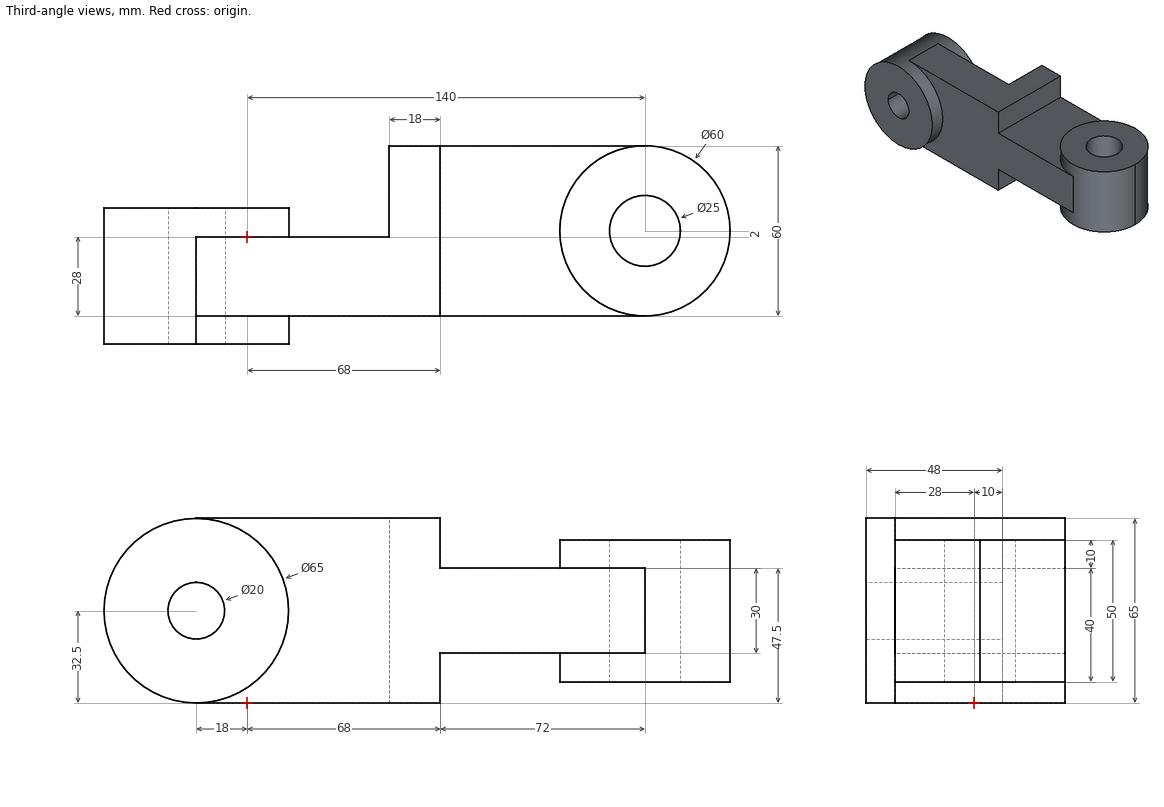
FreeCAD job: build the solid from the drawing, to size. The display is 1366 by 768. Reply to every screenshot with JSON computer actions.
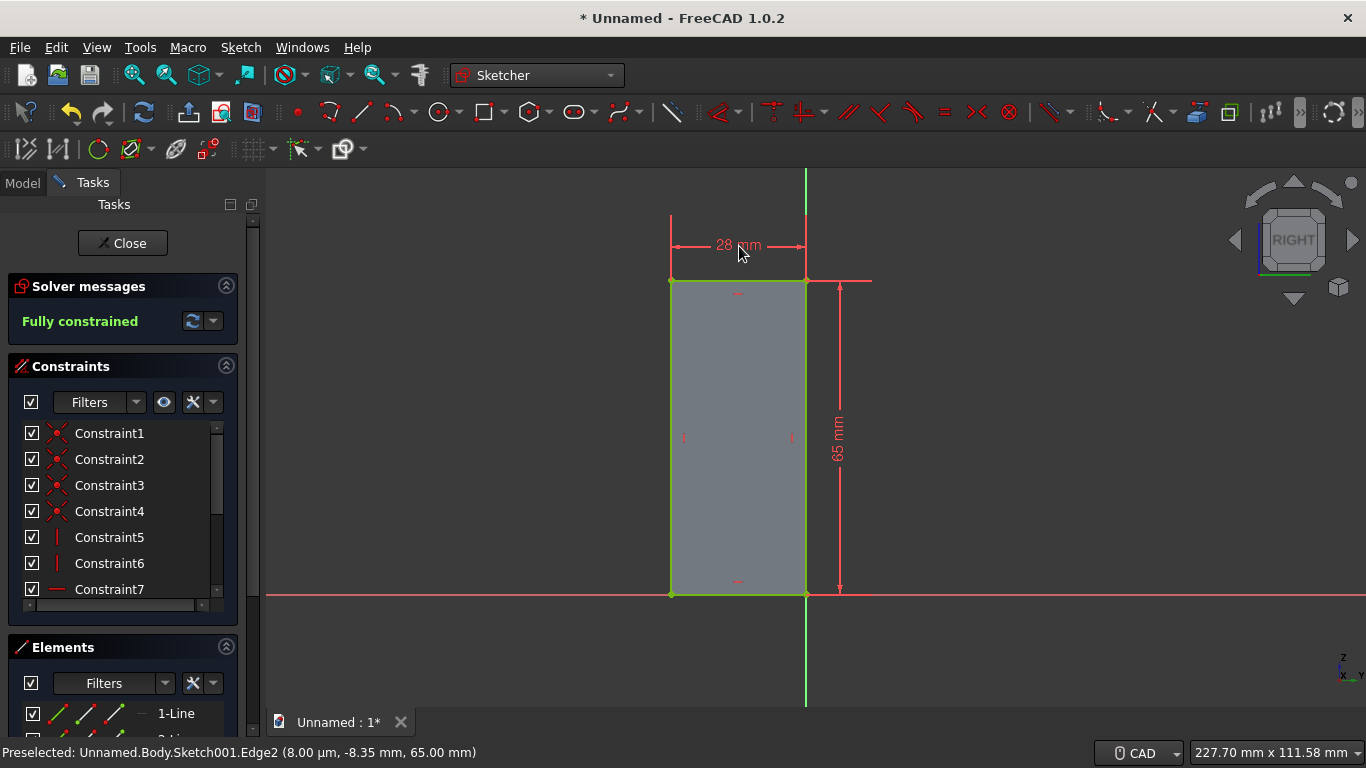
{"action": "left_click", "coordinate": [123, 243]}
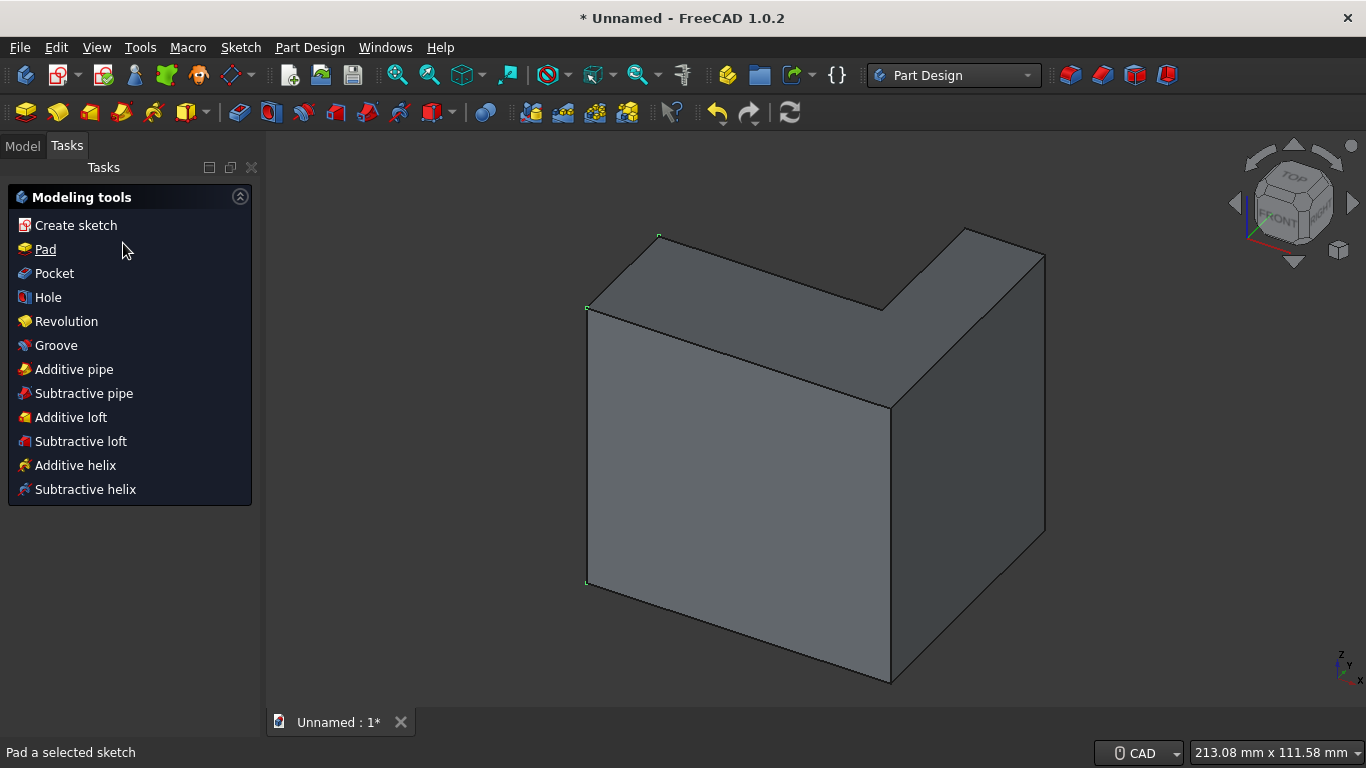
{"action": "left_click", "coordinate": [26, 112]}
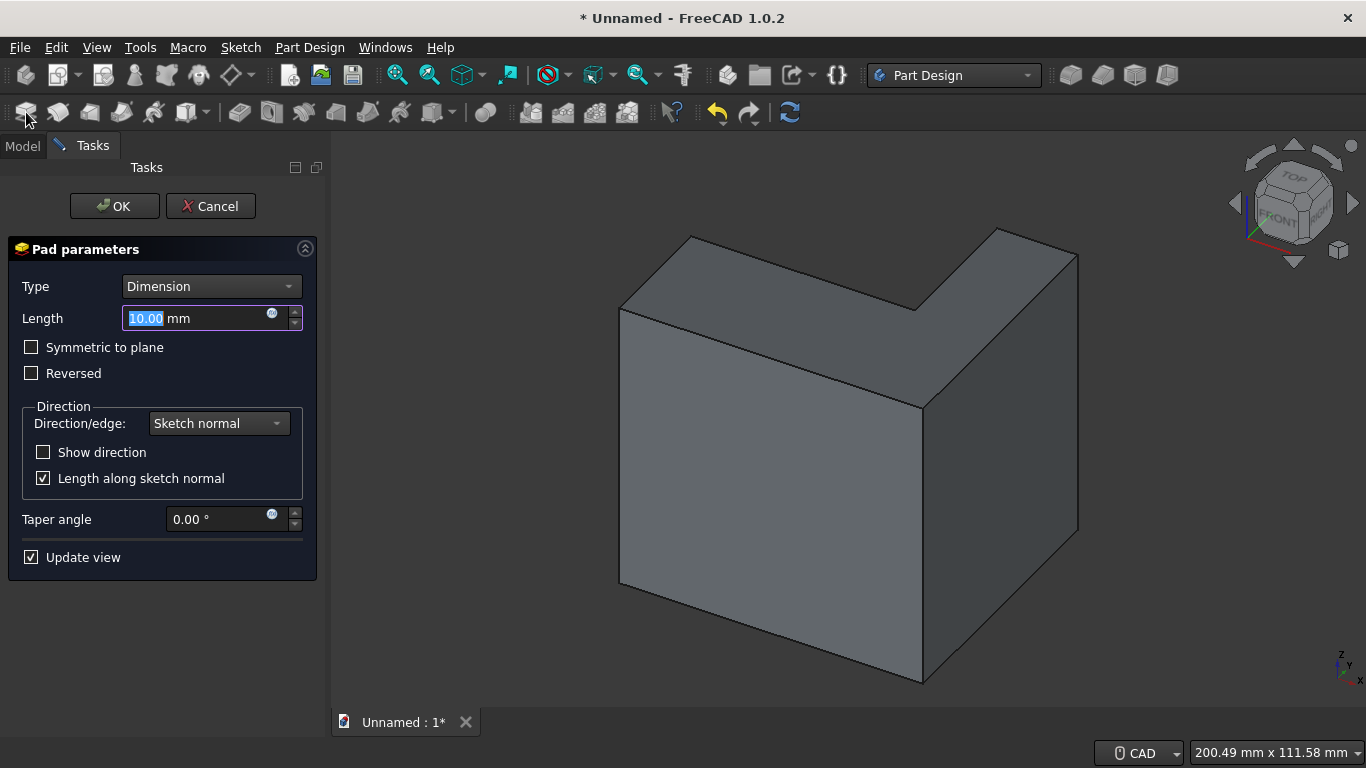
{"action": "type", "text": "18"}
{"action": "key", "text": "Tab"}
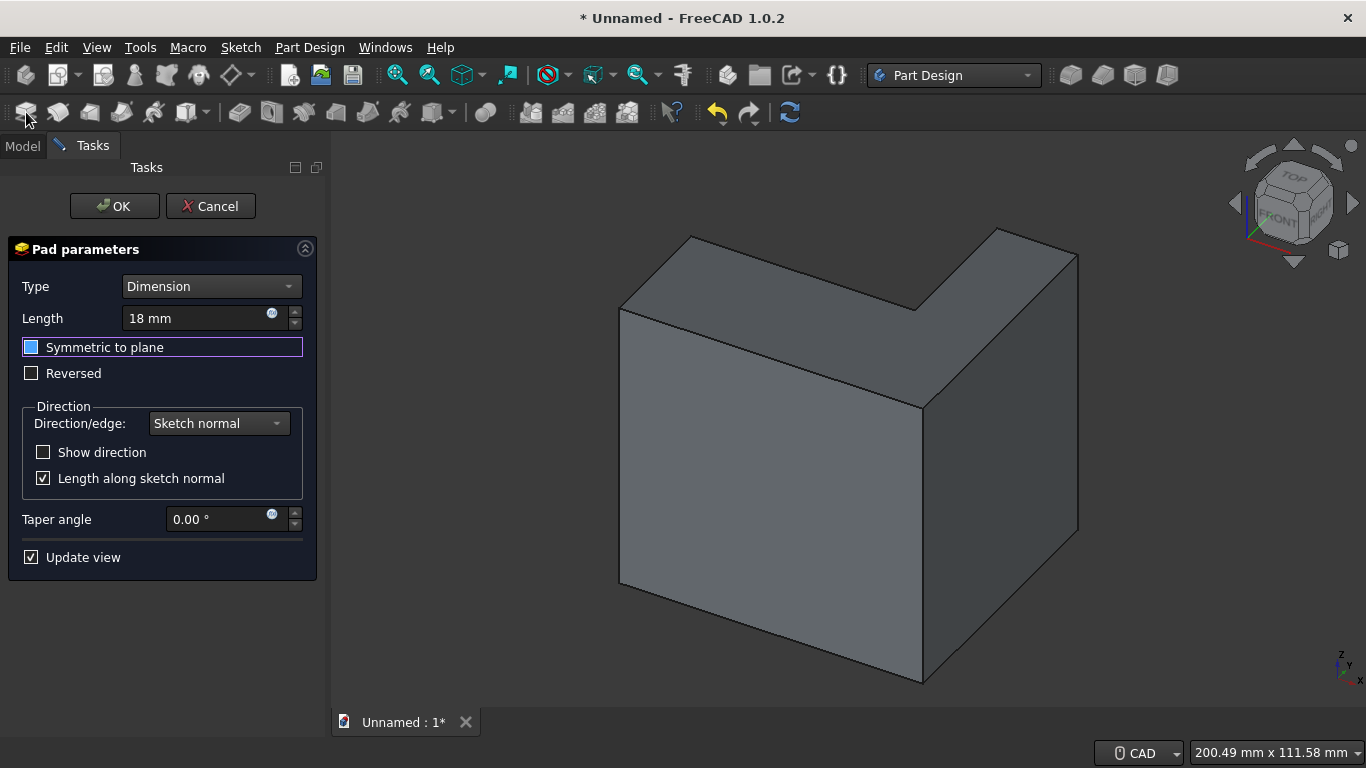
{"action": "left_click", "coordinate": [30, 373]}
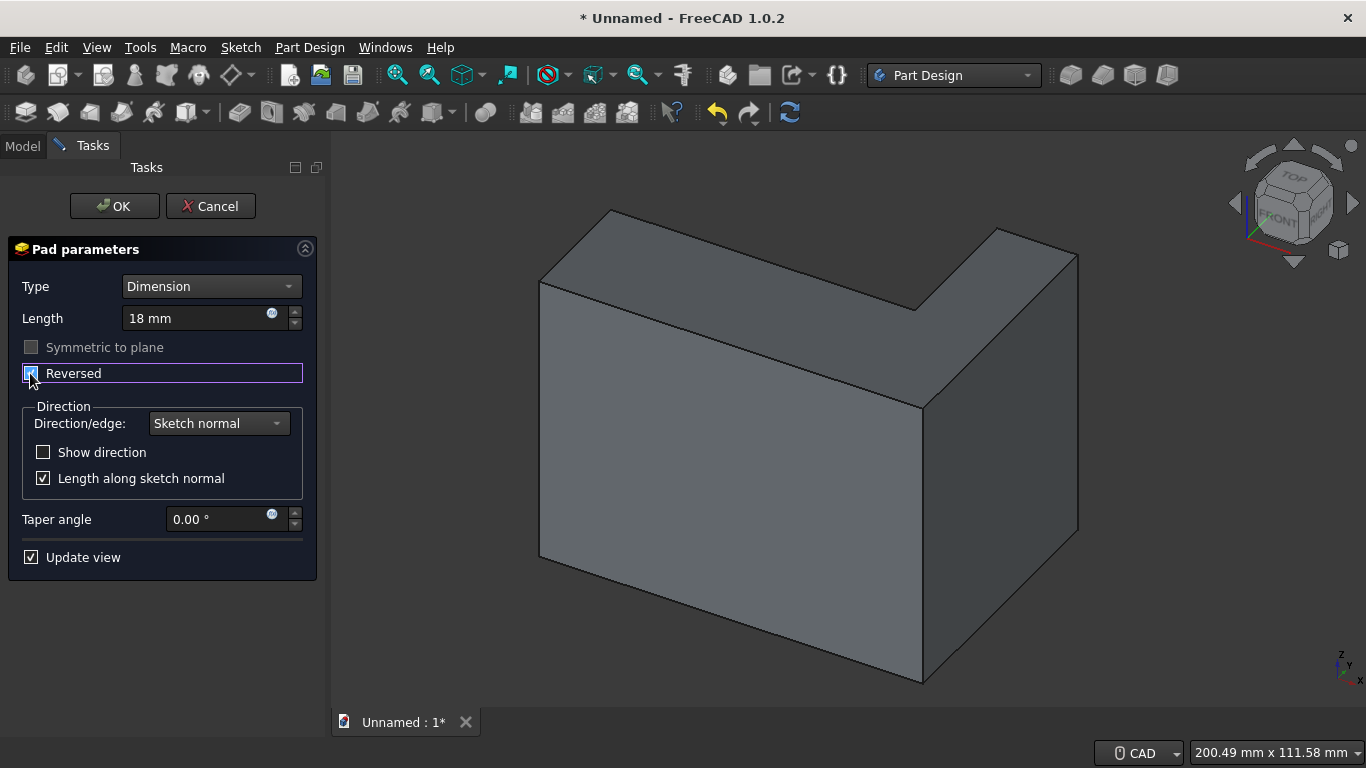
{"action": "left_click", "coordinate": [115, 206]}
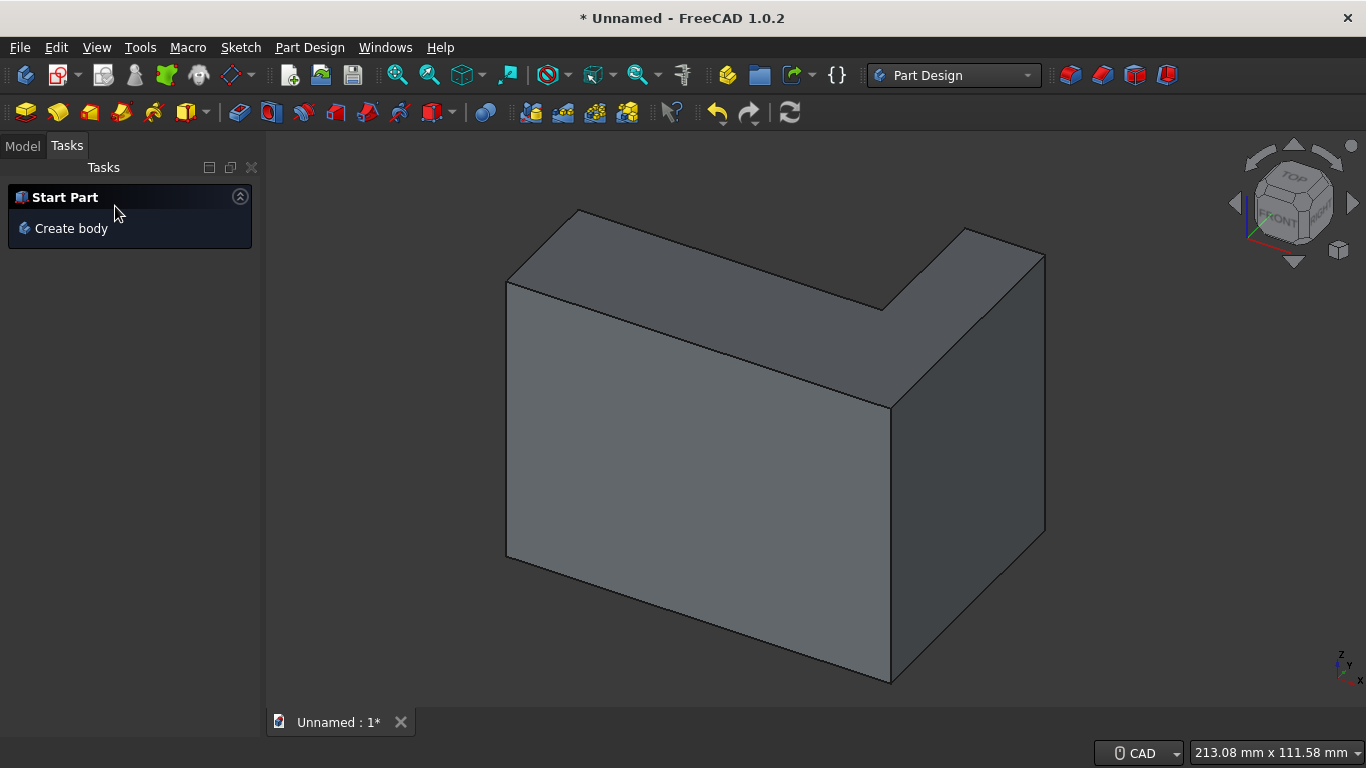
{"action": "key", "text": "v f"}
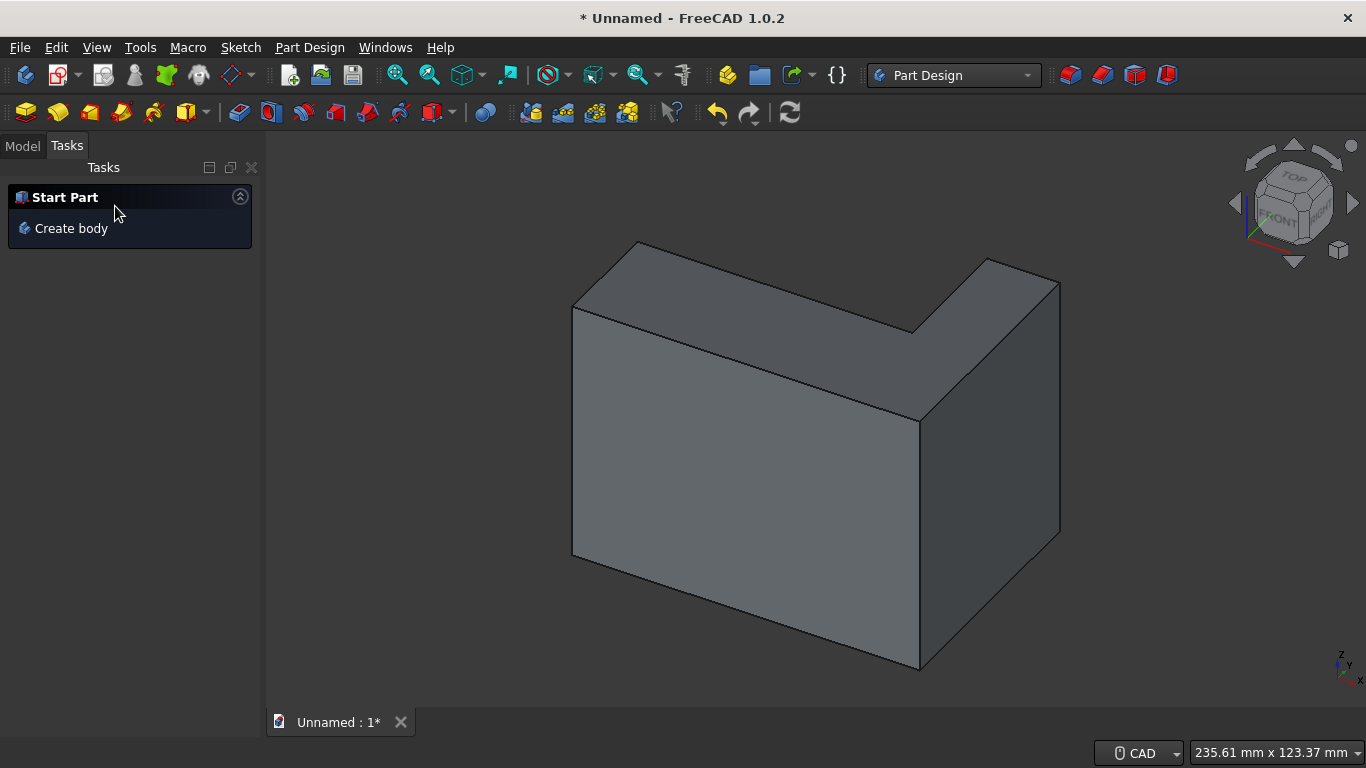
{"action": "key", "text": "4"}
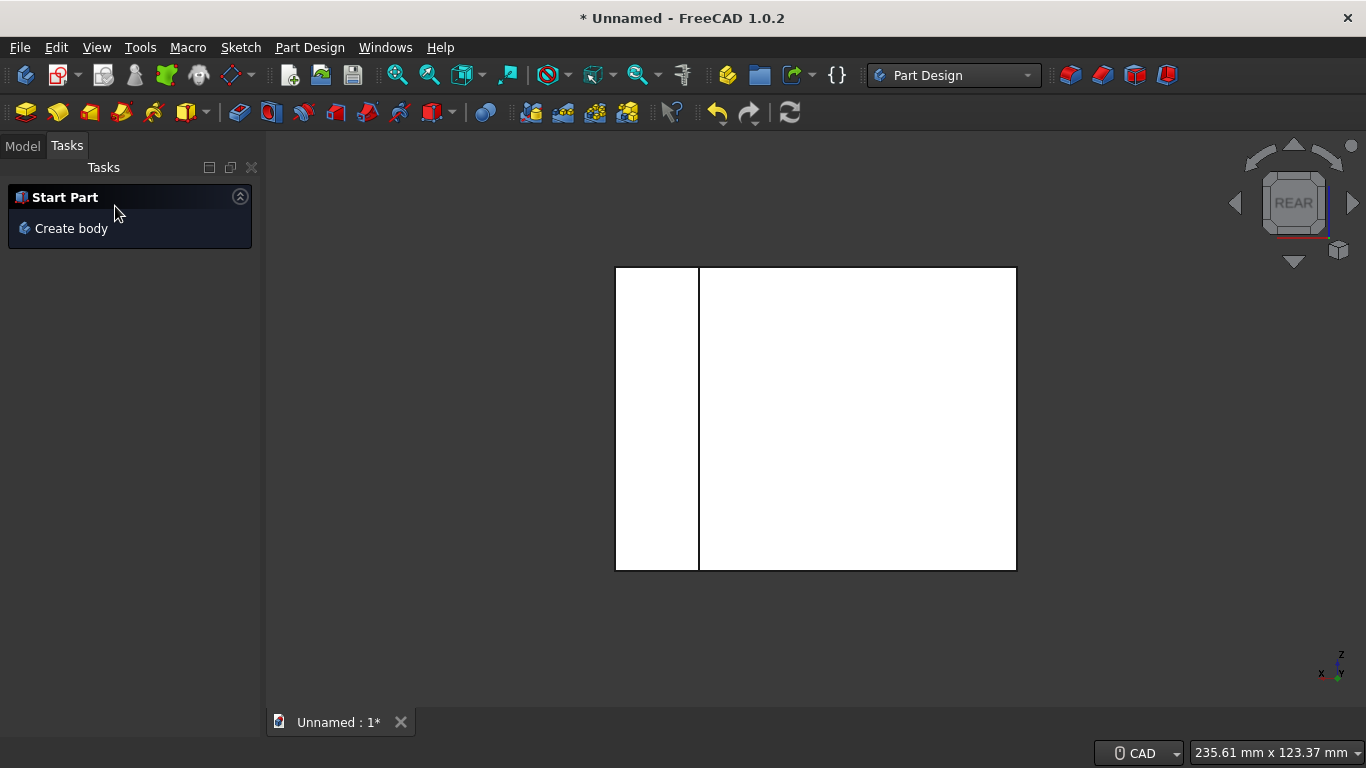
{"action": "left_click", "coordinate": [858, 418]}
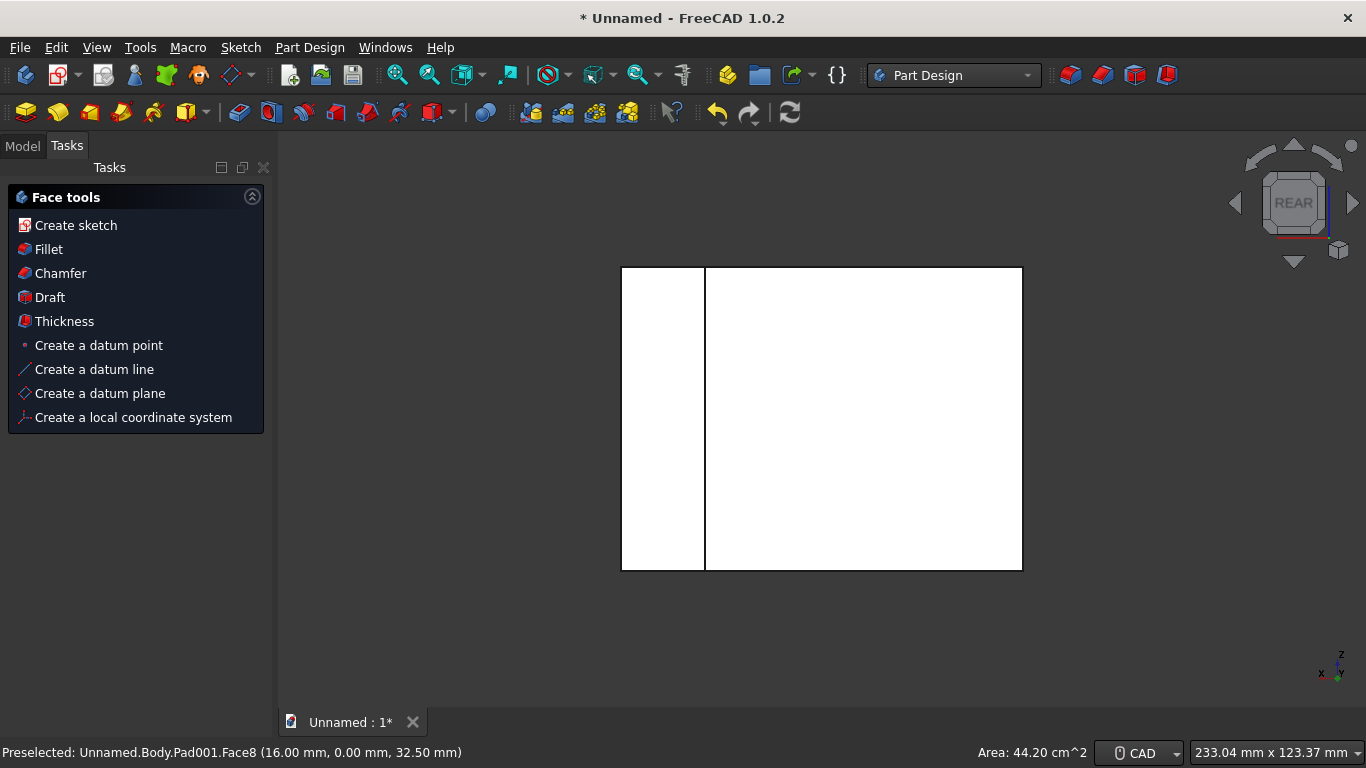
{"action": "left_click", "coordinate": [58, 76]}